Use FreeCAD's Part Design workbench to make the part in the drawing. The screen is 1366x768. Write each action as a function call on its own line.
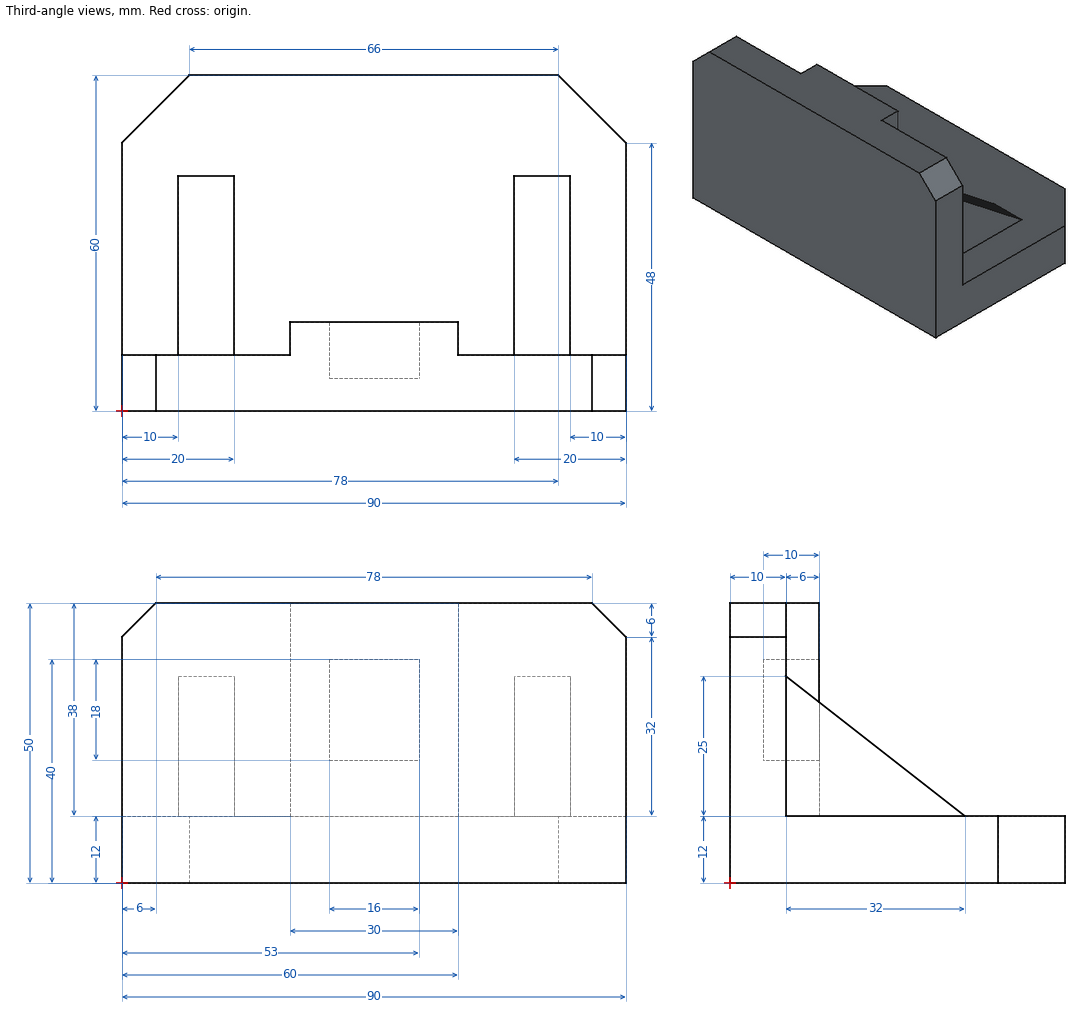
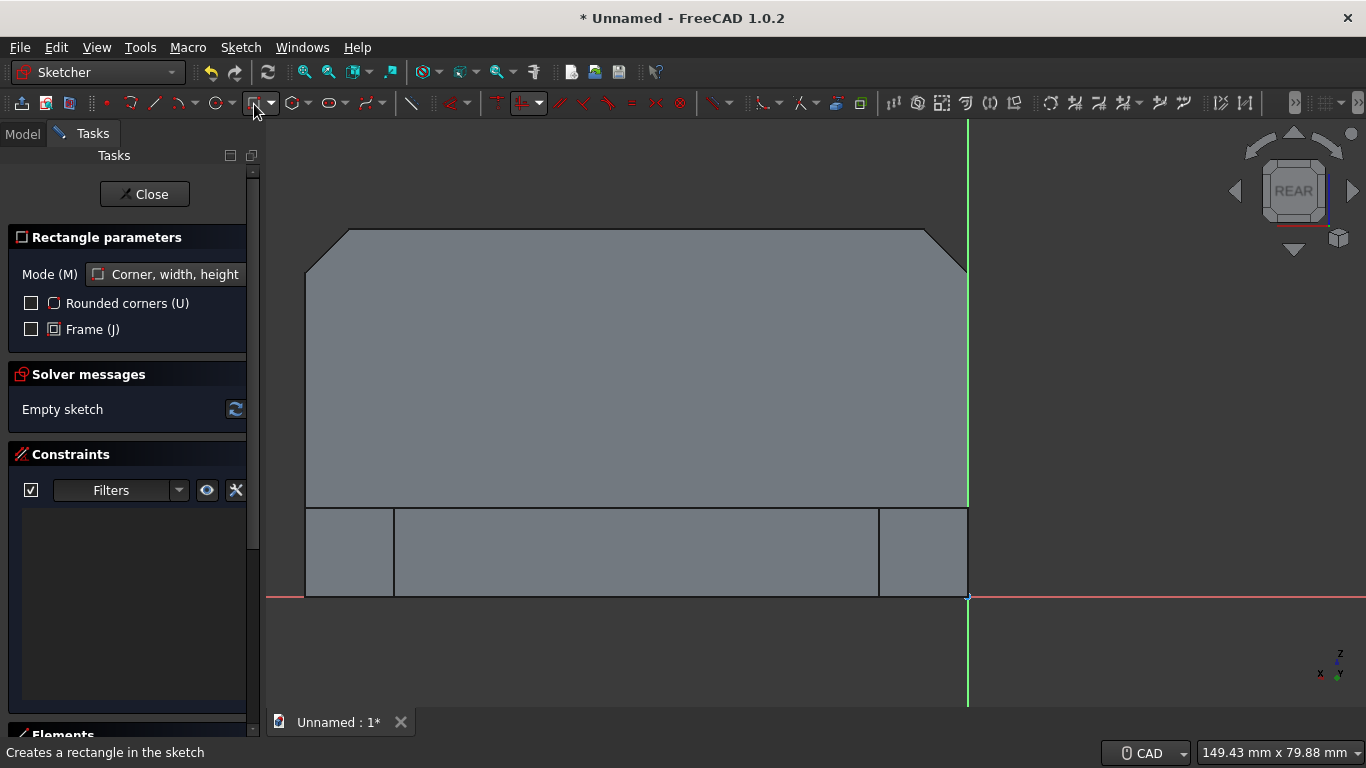
click(526, 229)
move(747, 508)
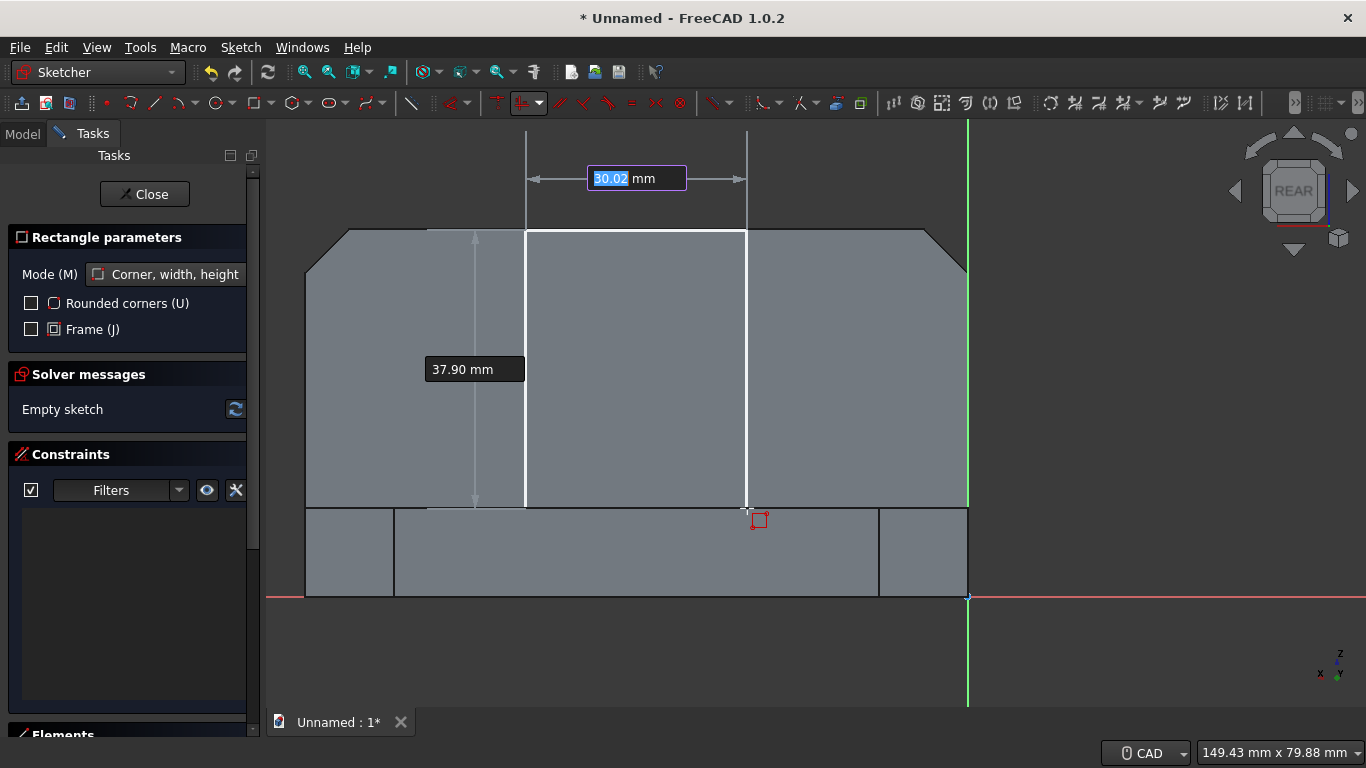
text(30)
key(Tab)
text(38)
key(Return)
key(Escape)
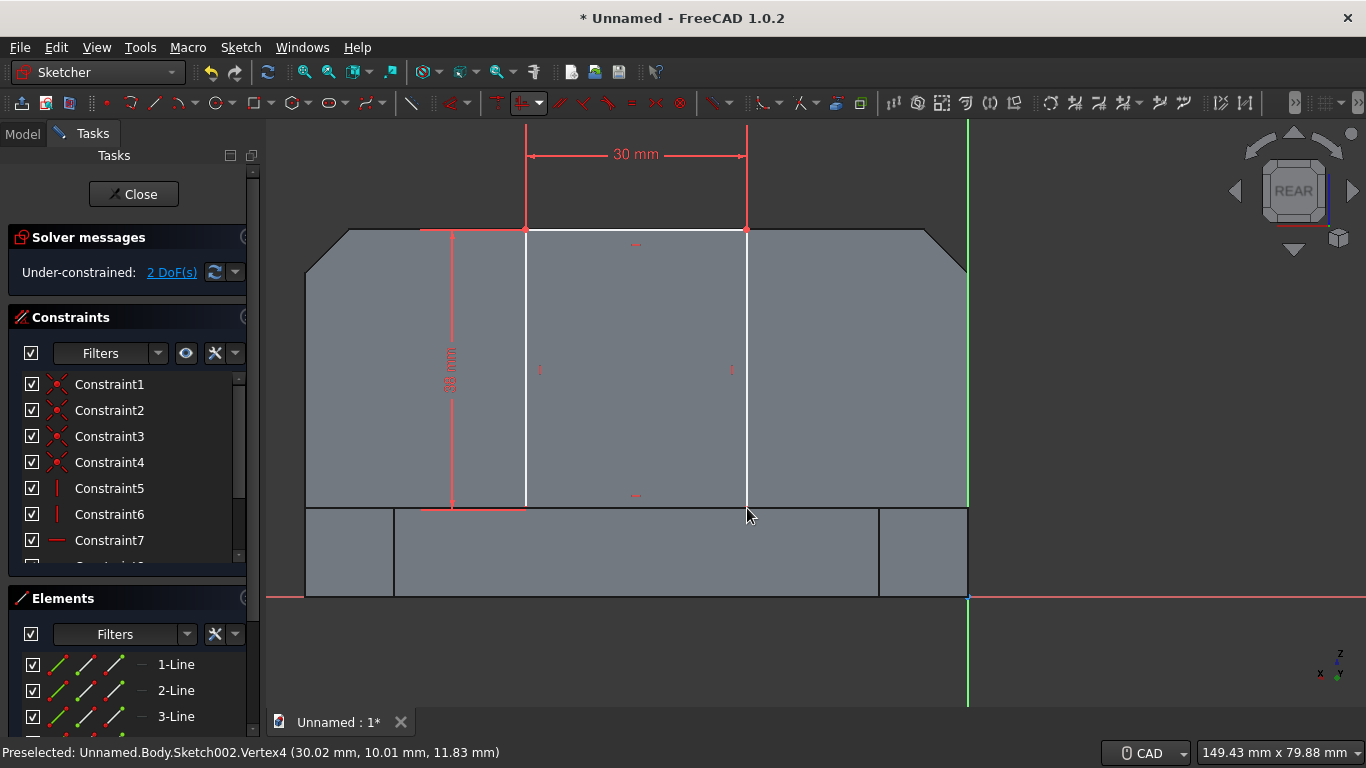
click(450, 104)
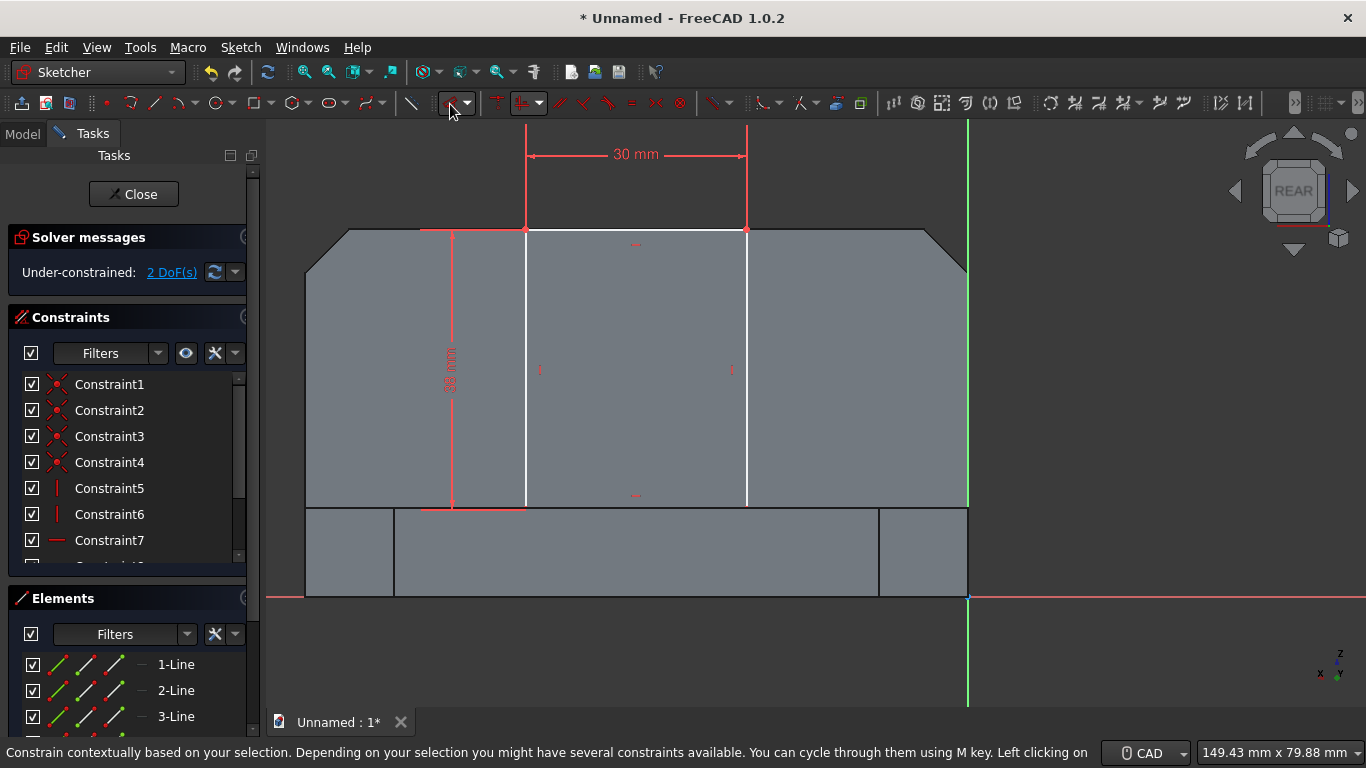
click(526, 230)
click(747, 631)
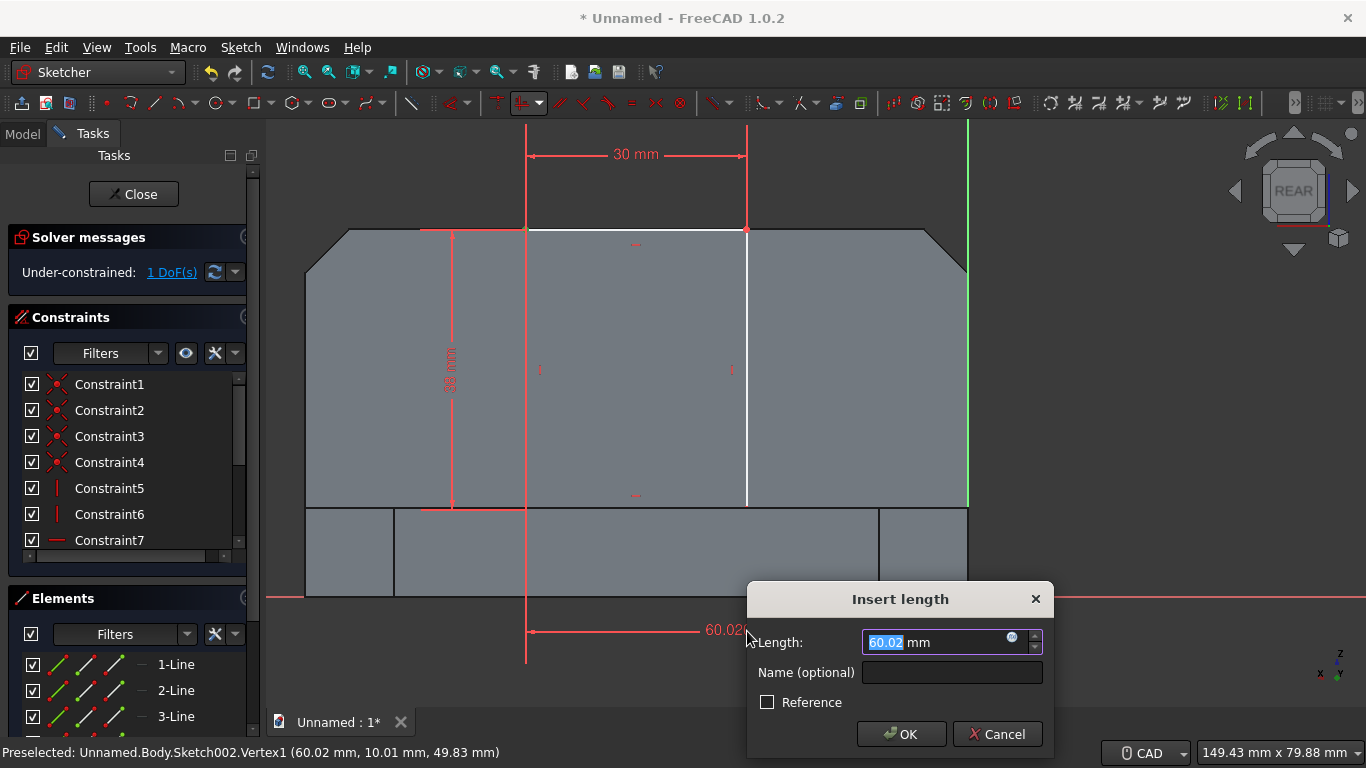
text(60)
key(Return)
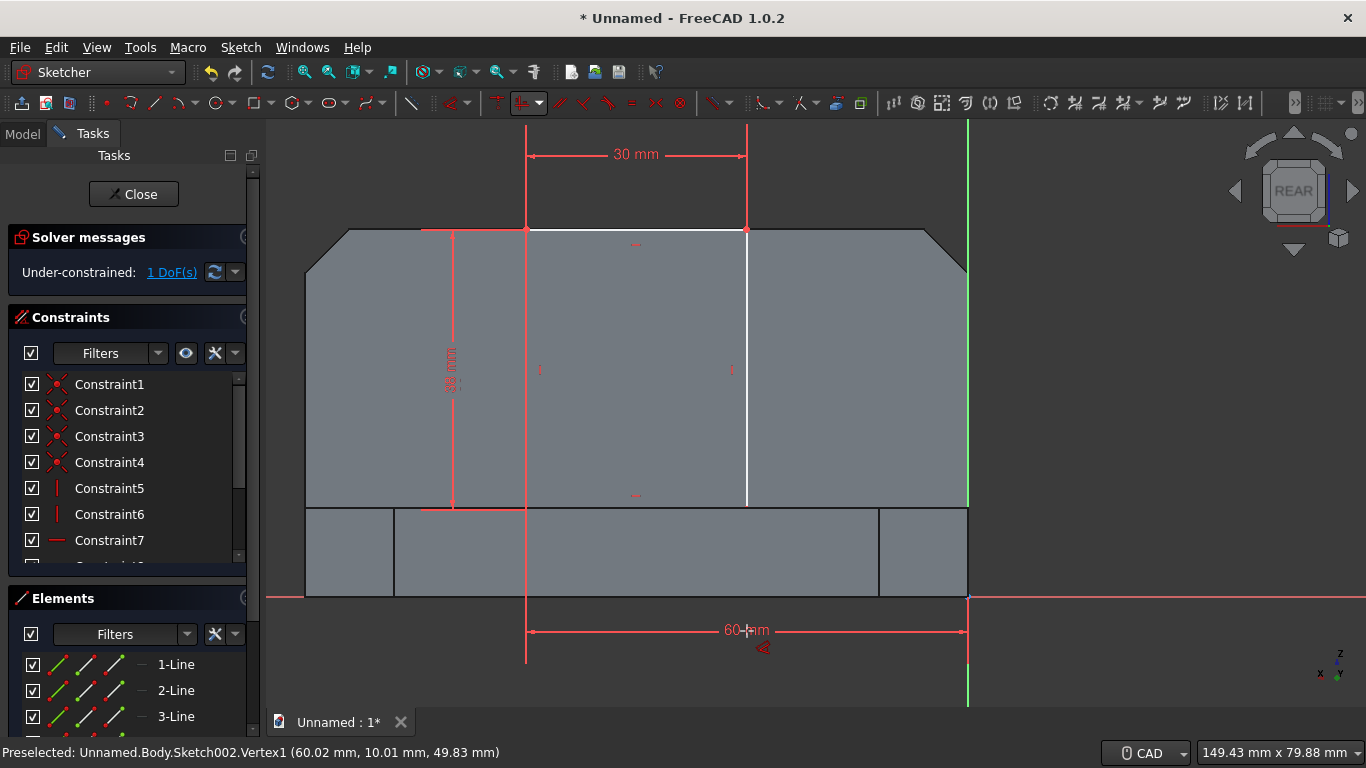
click(526, 230)
click(1002, 413)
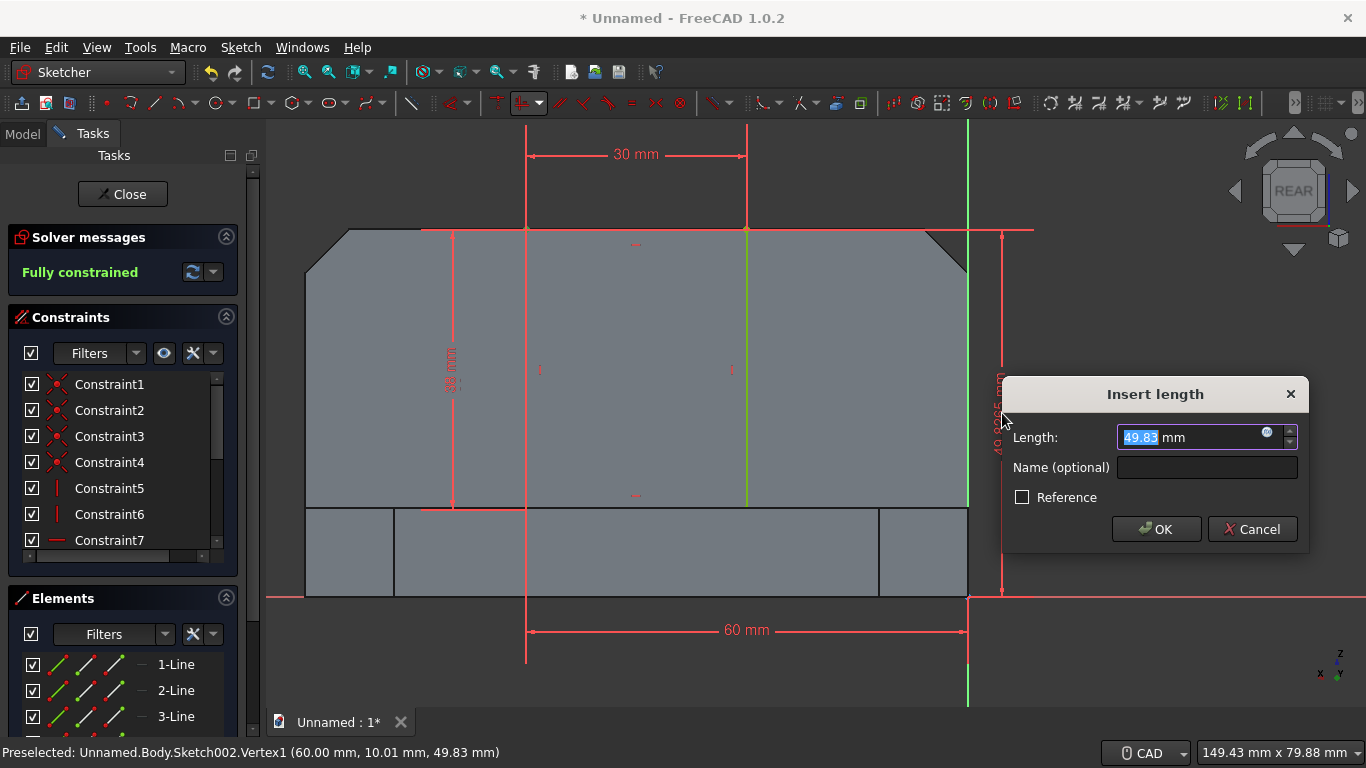
text(50)
key(Return)
key(Escape)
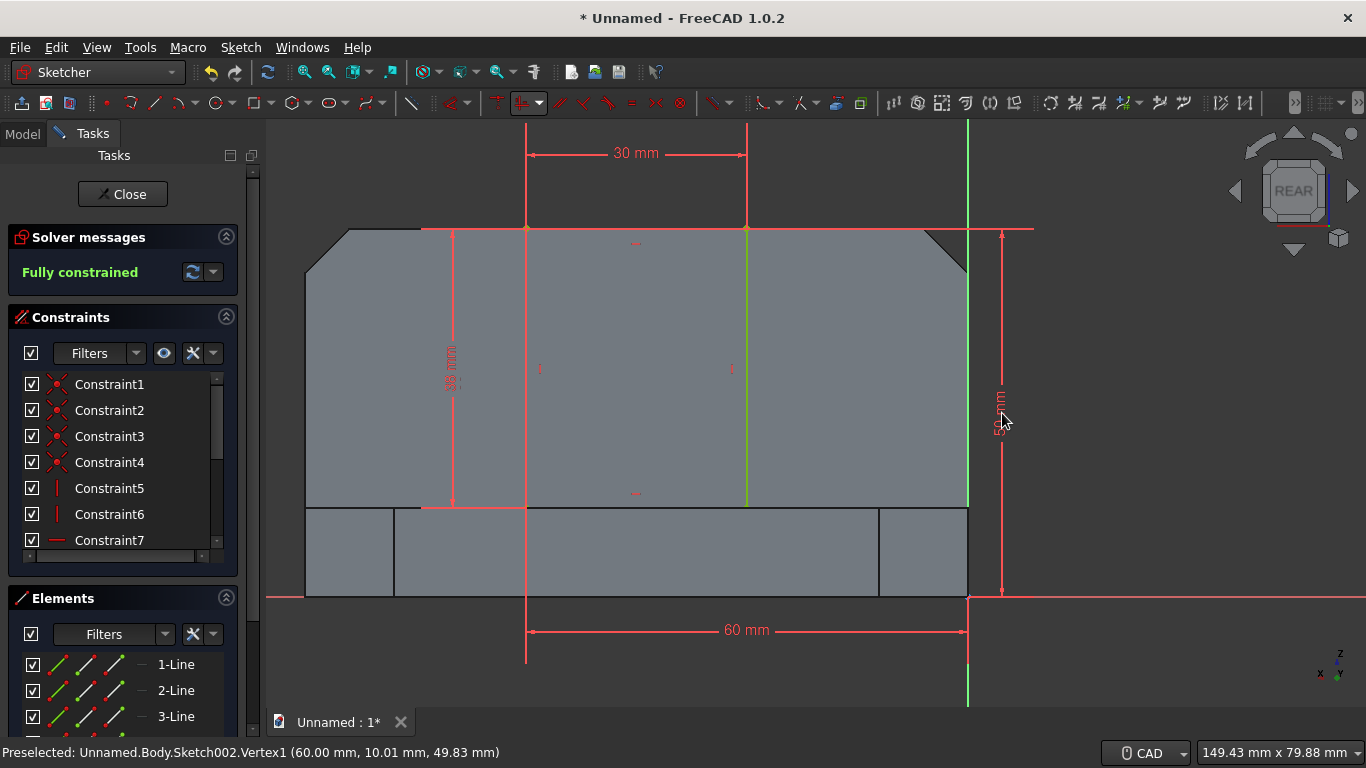
click(123, 194)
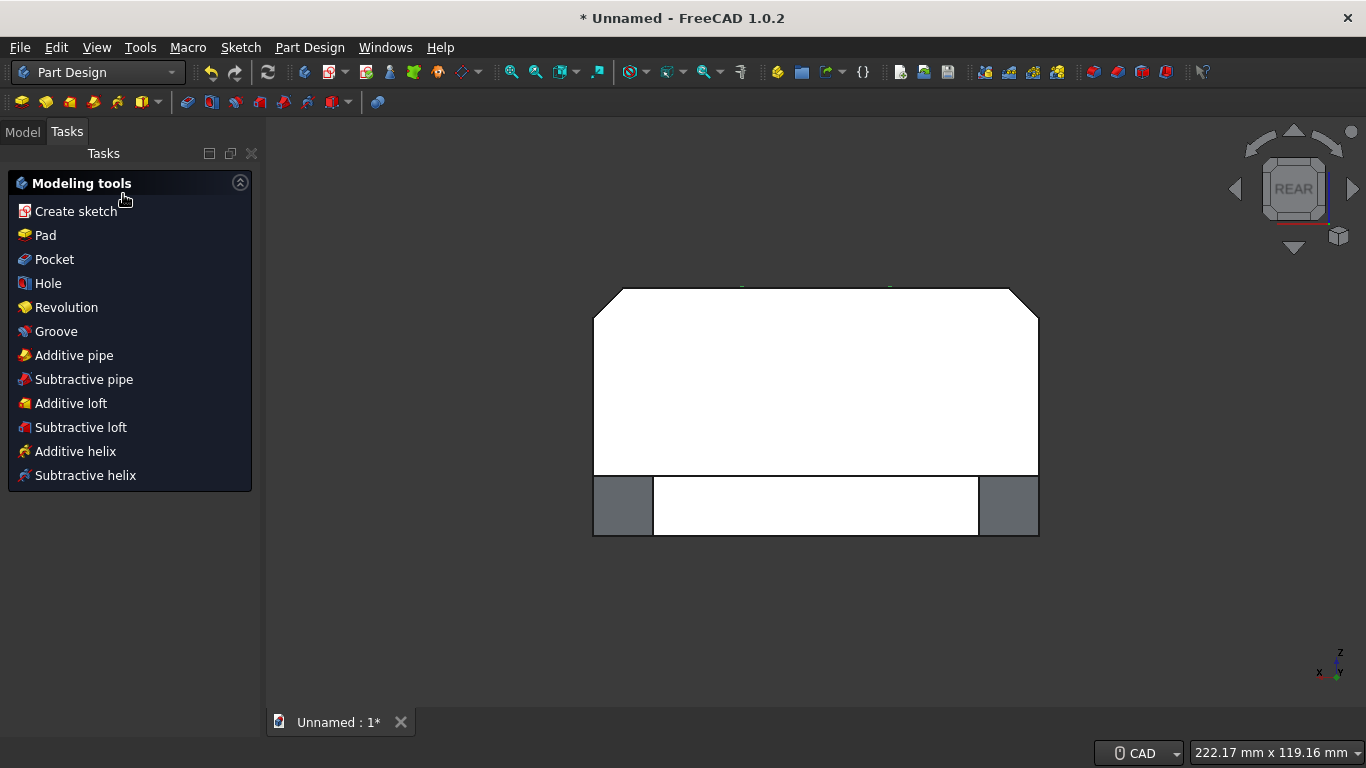
click(22, 102)